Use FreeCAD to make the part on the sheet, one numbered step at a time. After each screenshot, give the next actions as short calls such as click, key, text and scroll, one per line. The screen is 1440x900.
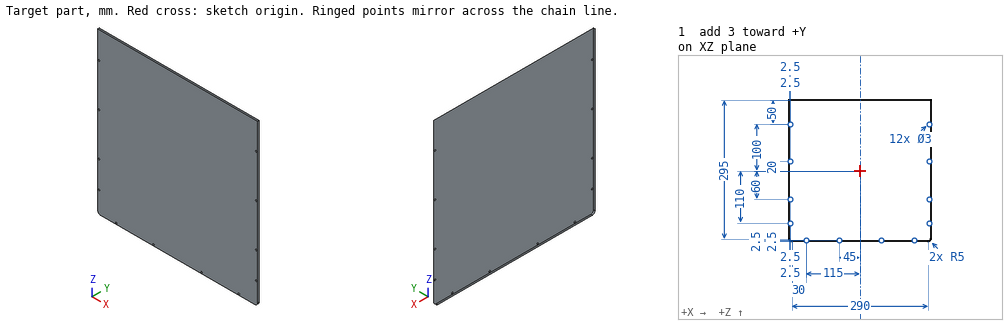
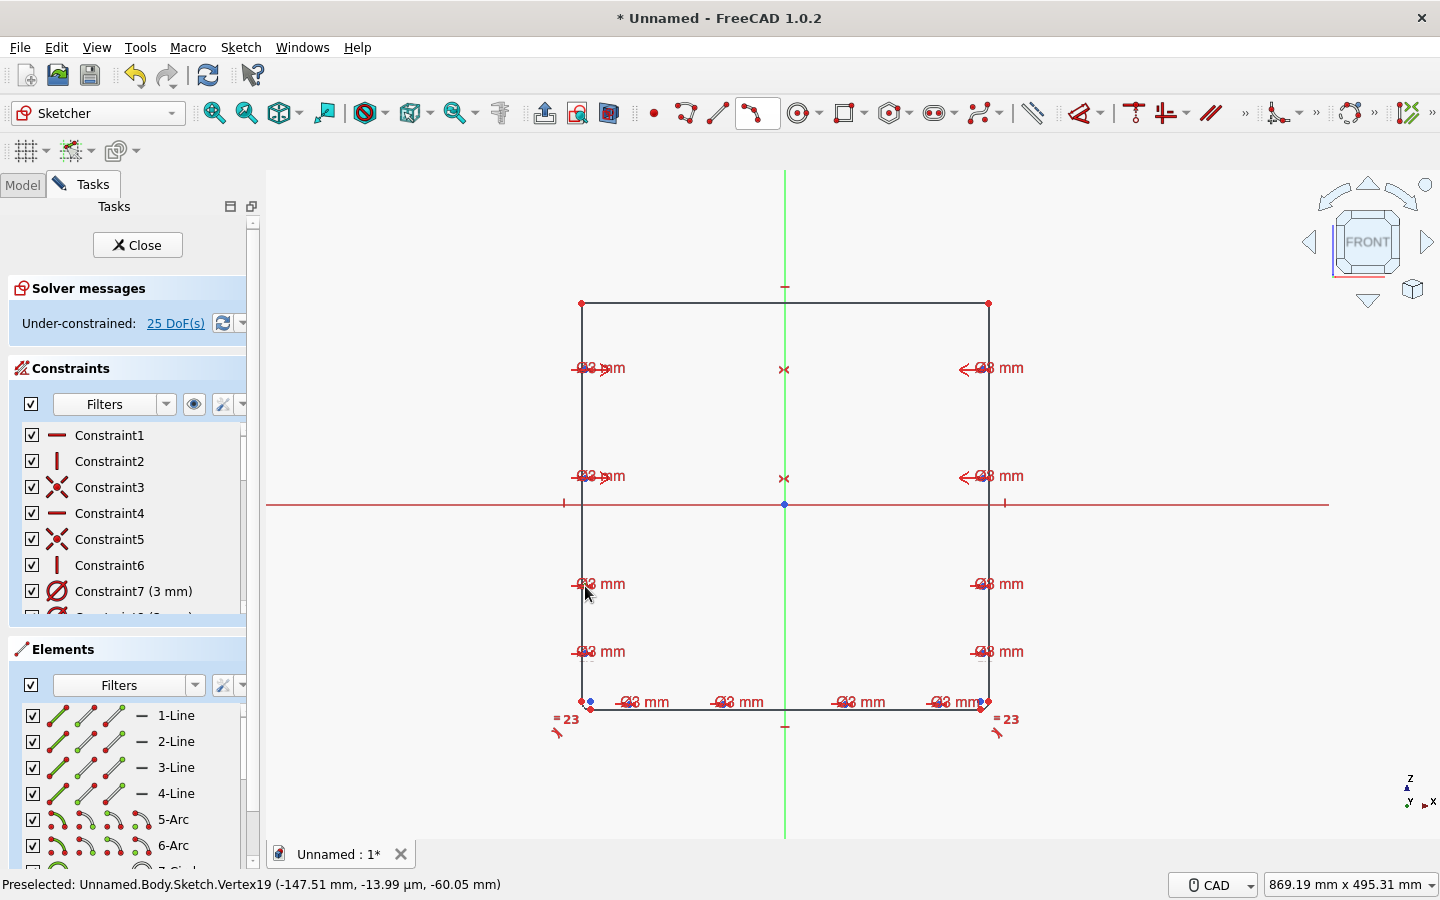
click(984, 586)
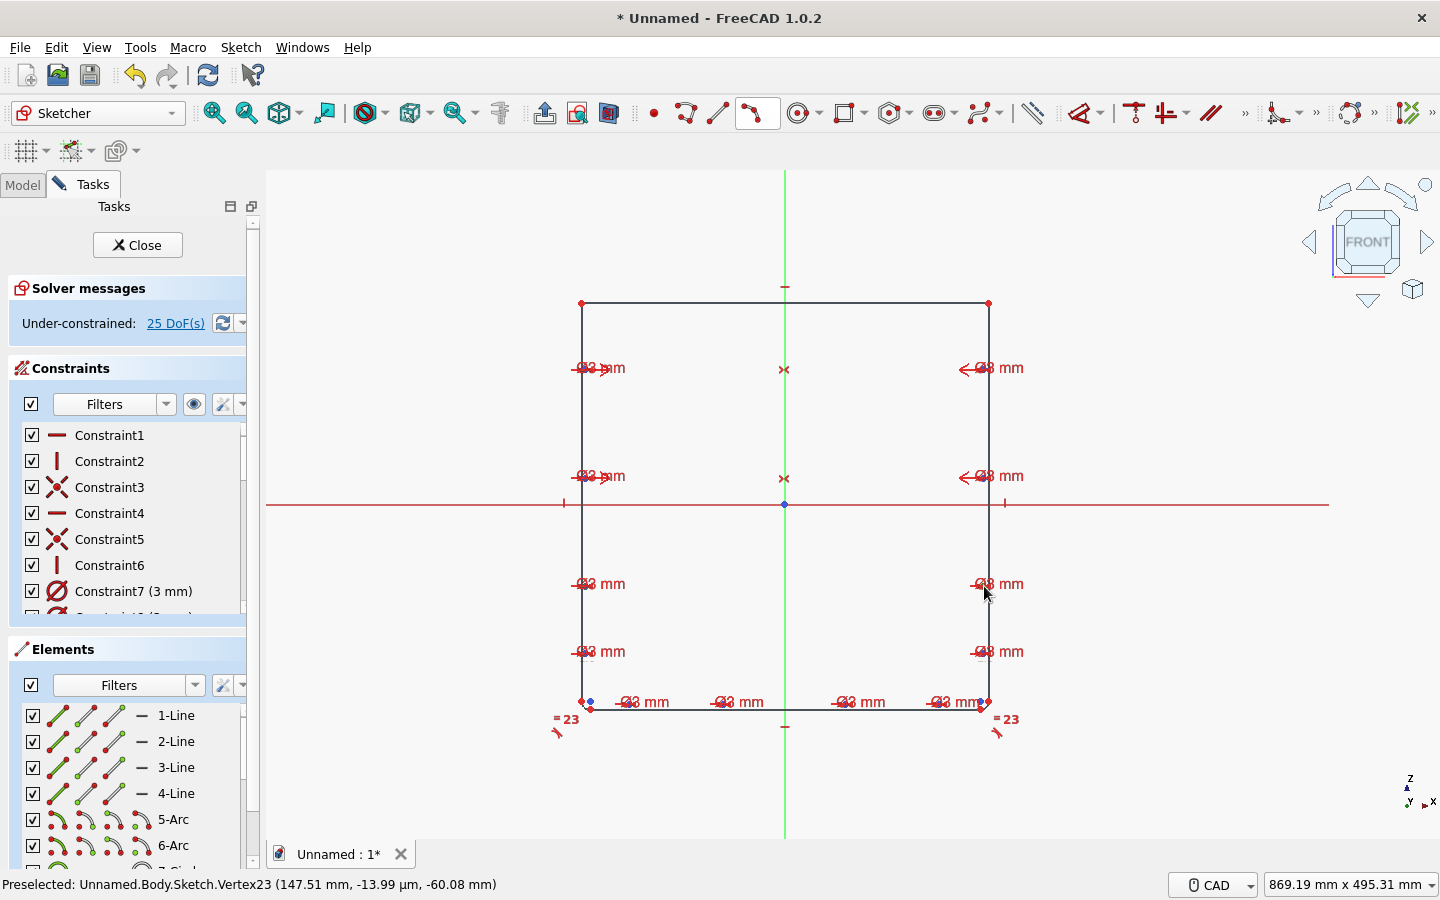
click(785, 767)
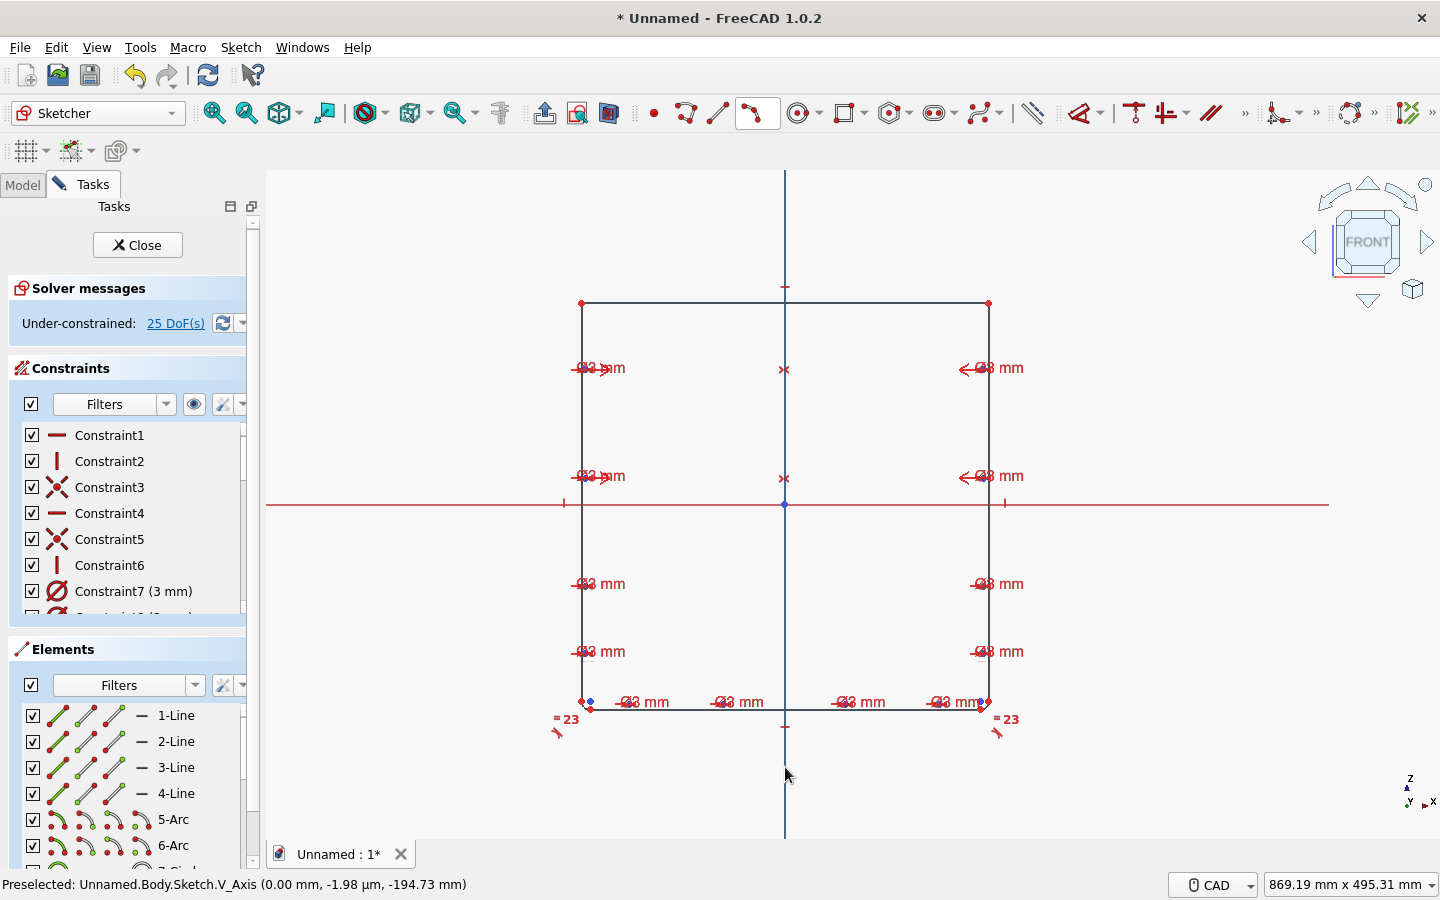
key(s)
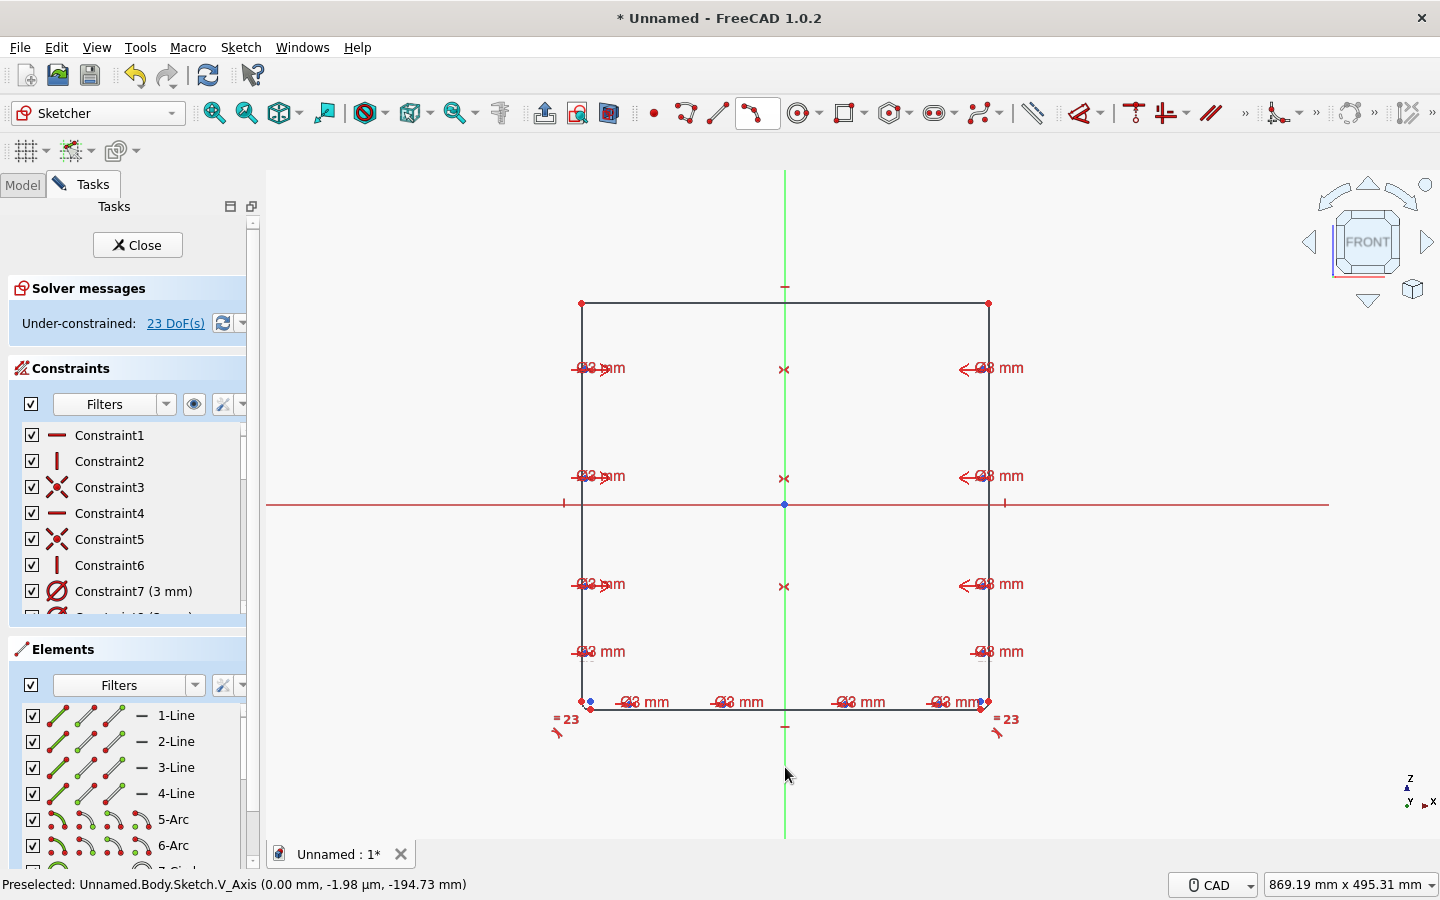
click(724, 704)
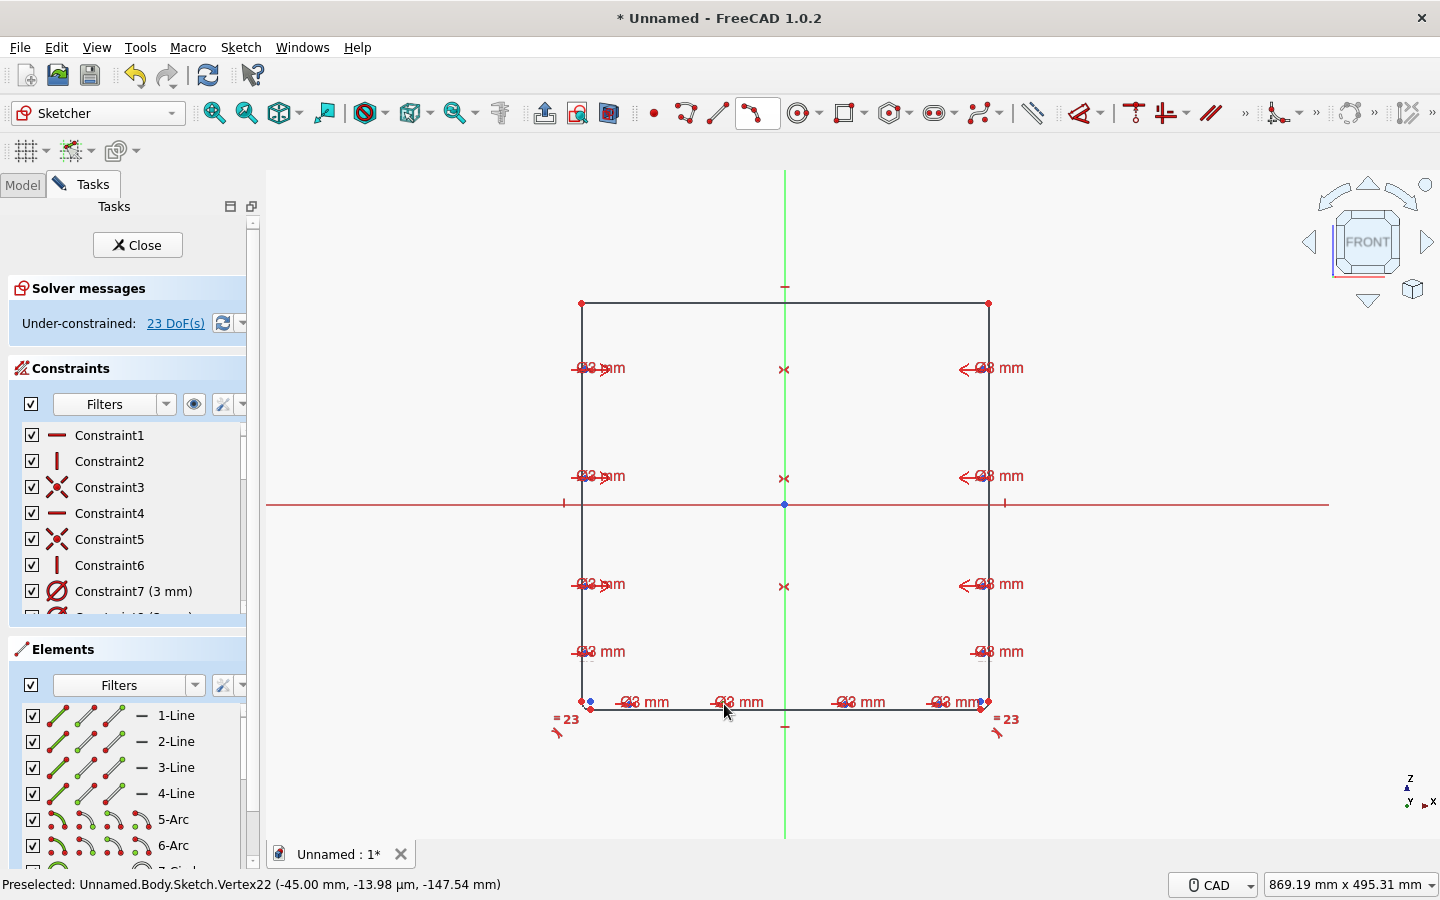
click(845, 704)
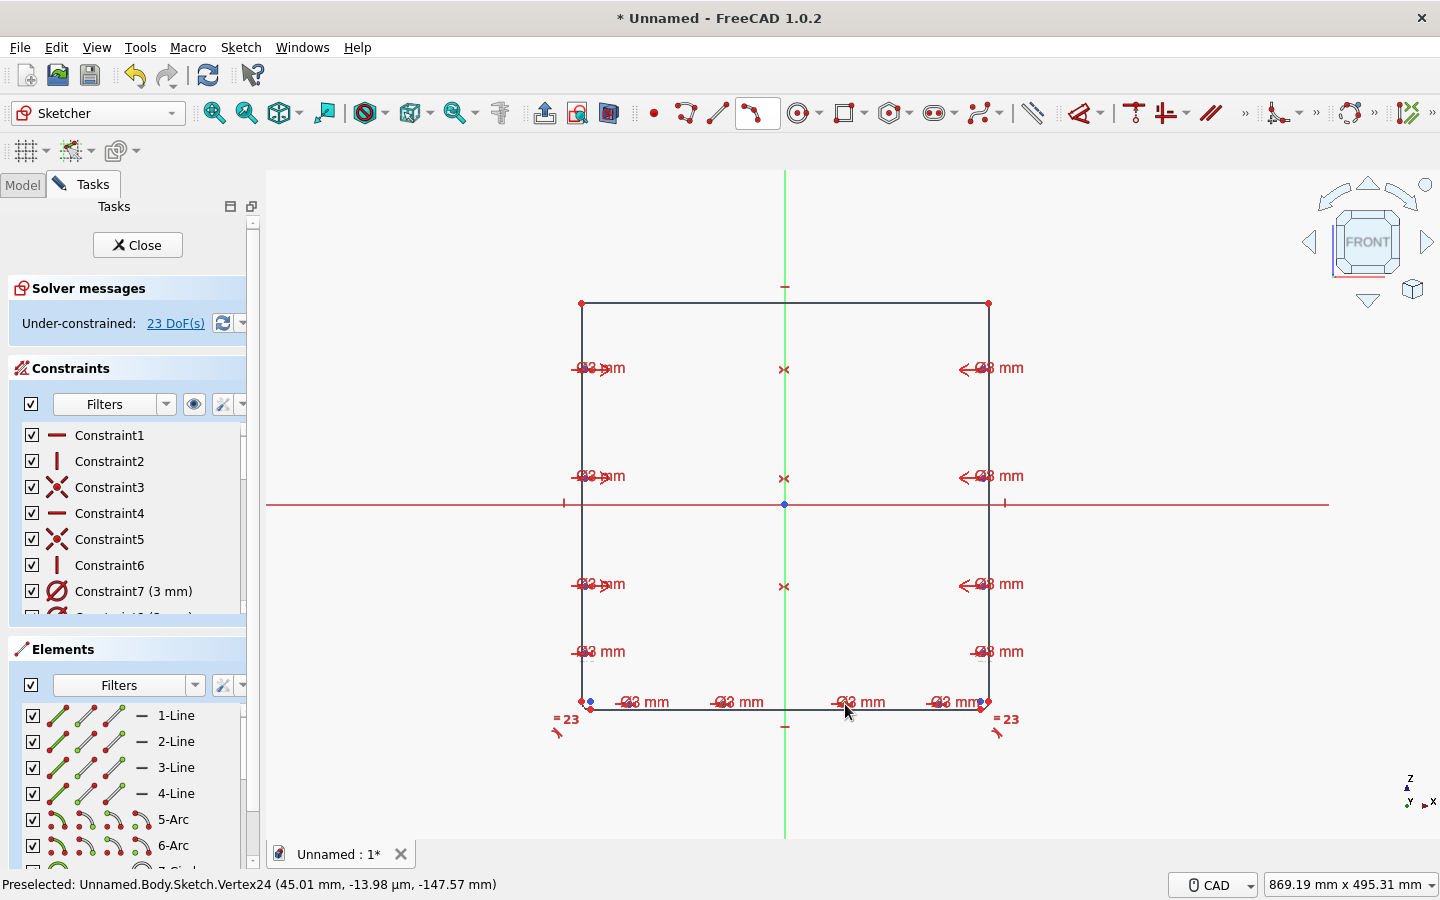
click(785, 767)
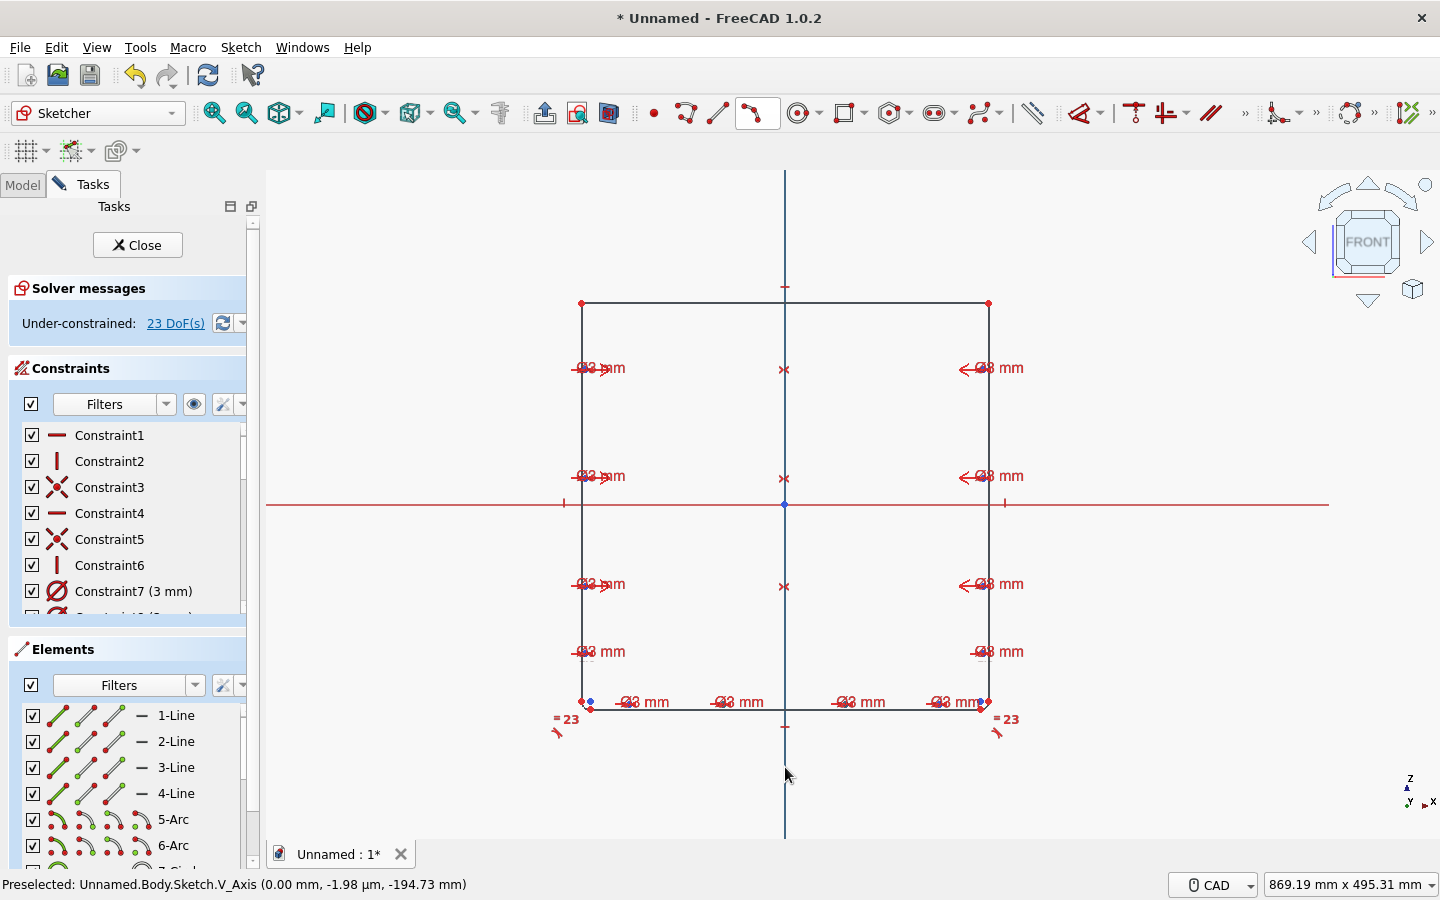
key(s)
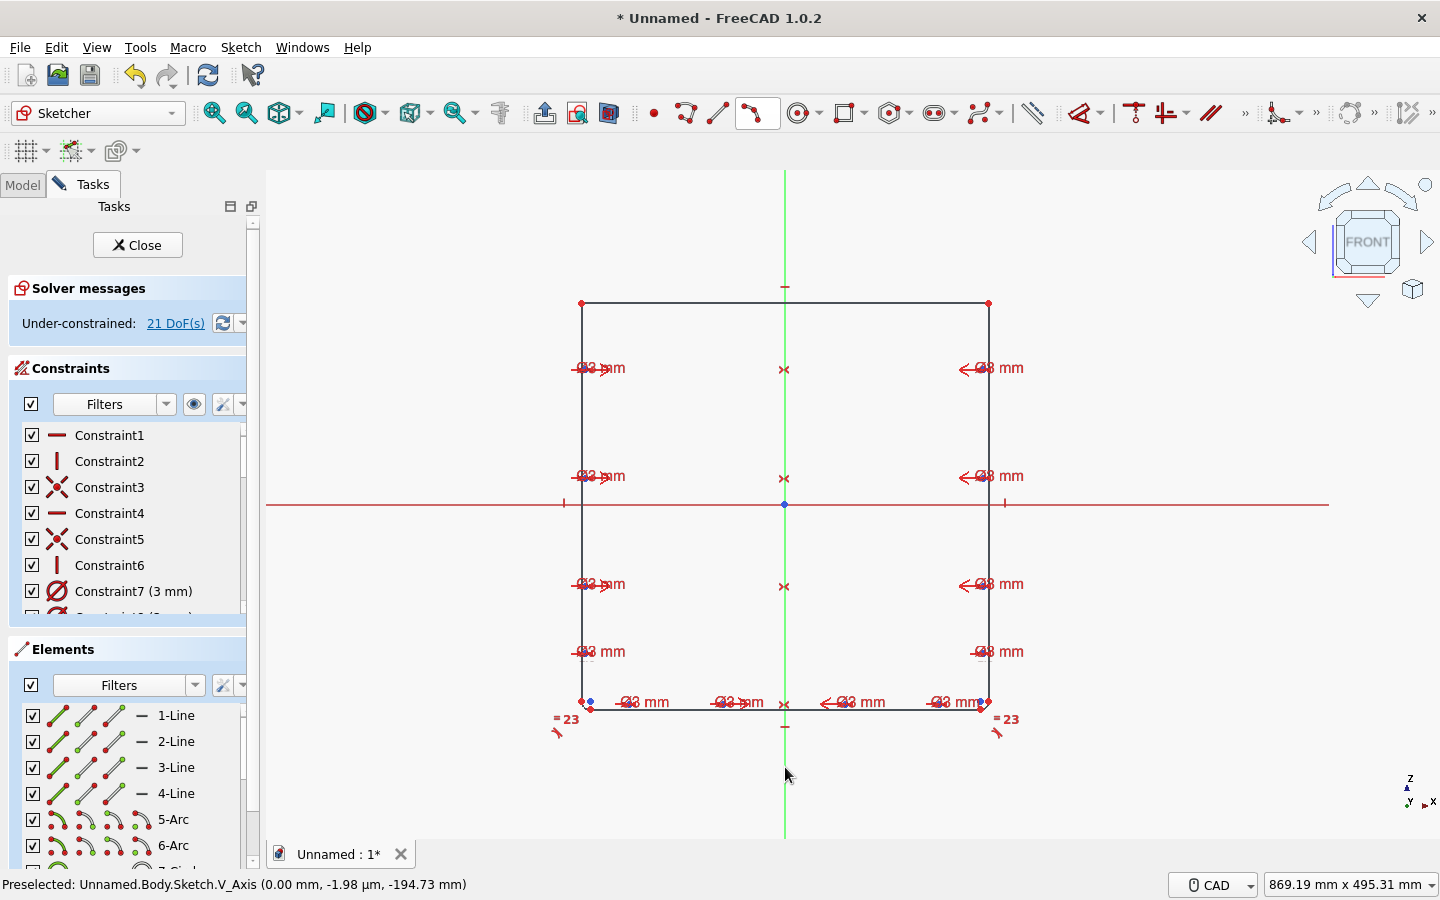
click(585, 654)